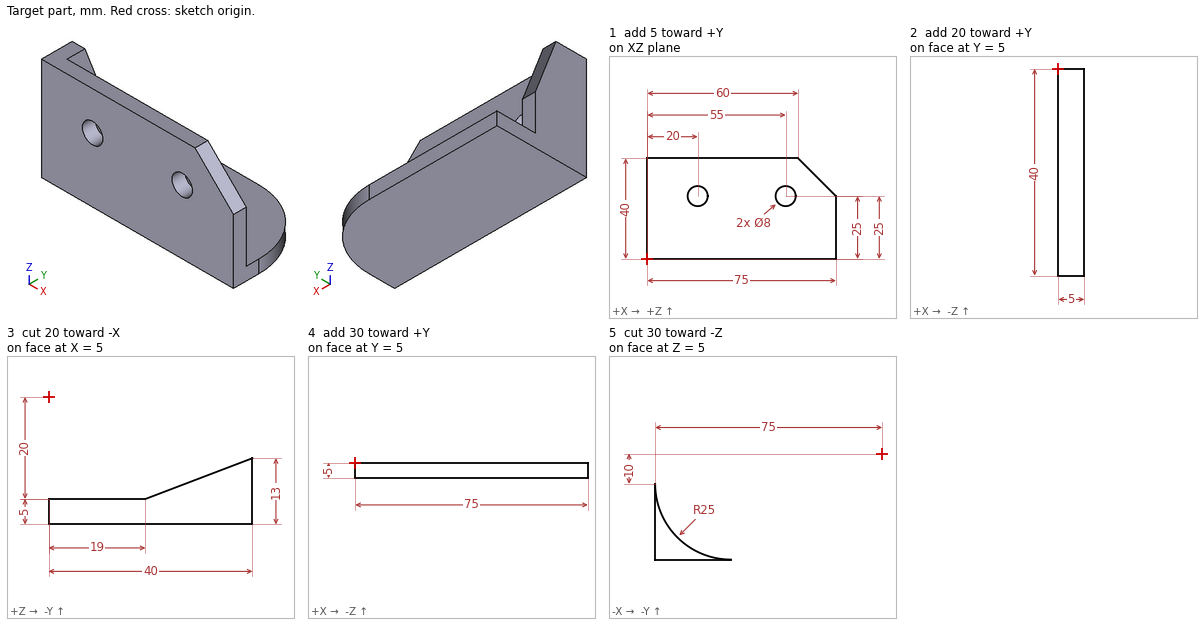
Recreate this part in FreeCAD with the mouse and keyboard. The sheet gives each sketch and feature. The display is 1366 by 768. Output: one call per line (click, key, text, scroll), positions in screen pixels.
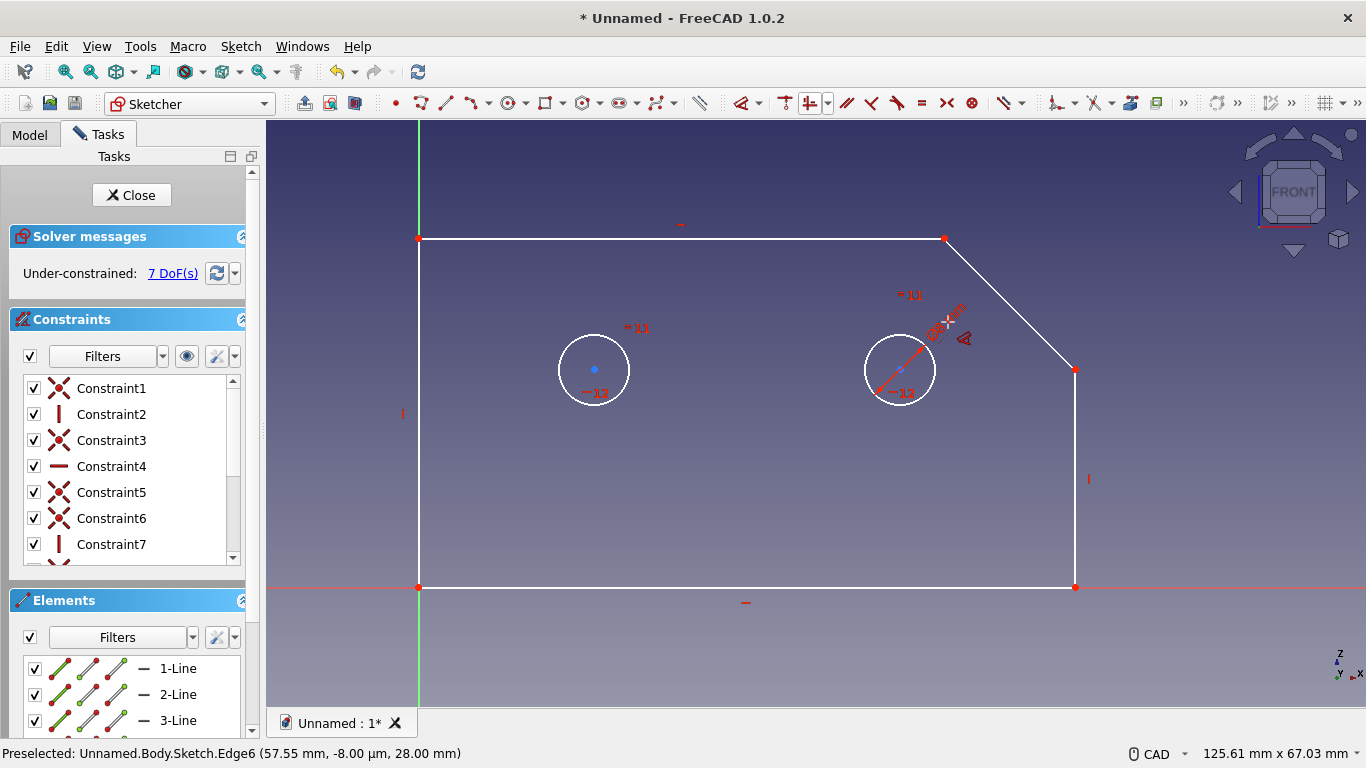
click(419, 483)
click(385, 413)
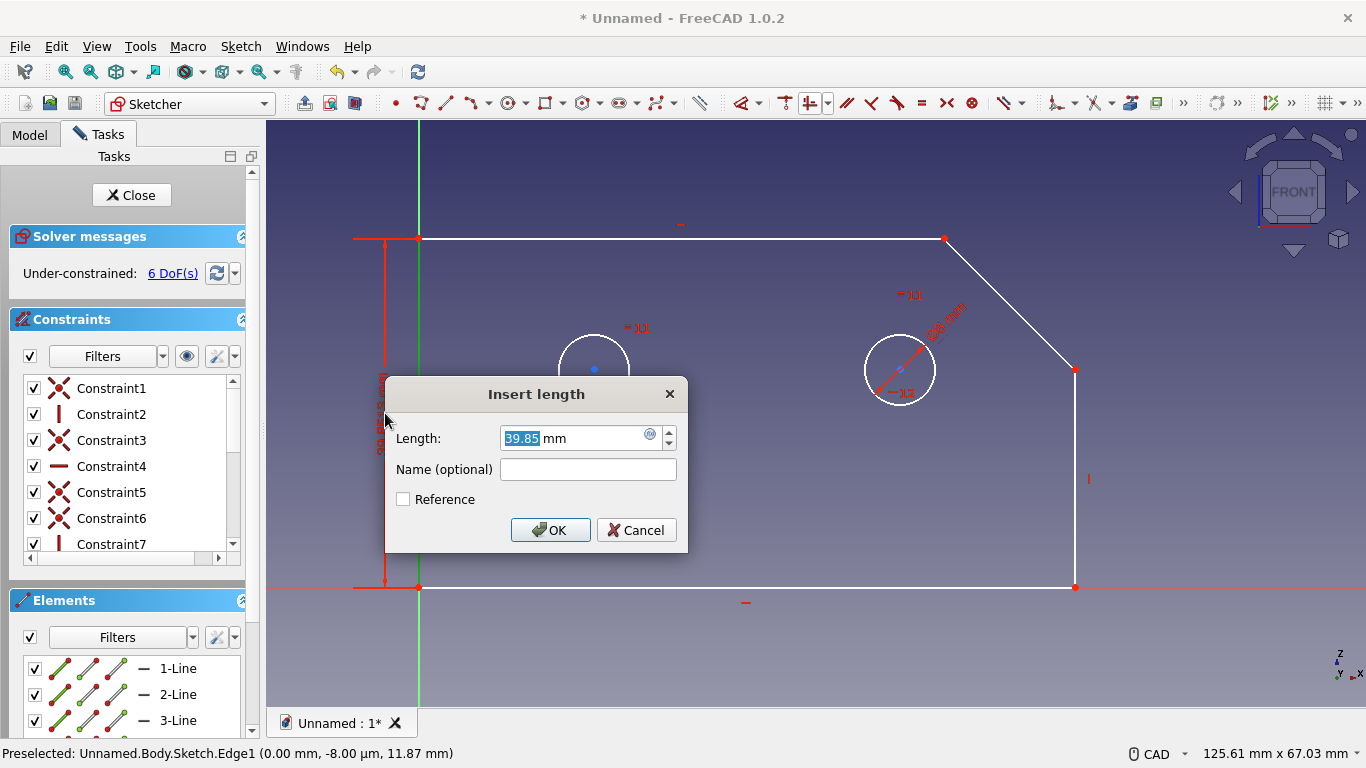
text(40)
key(Return)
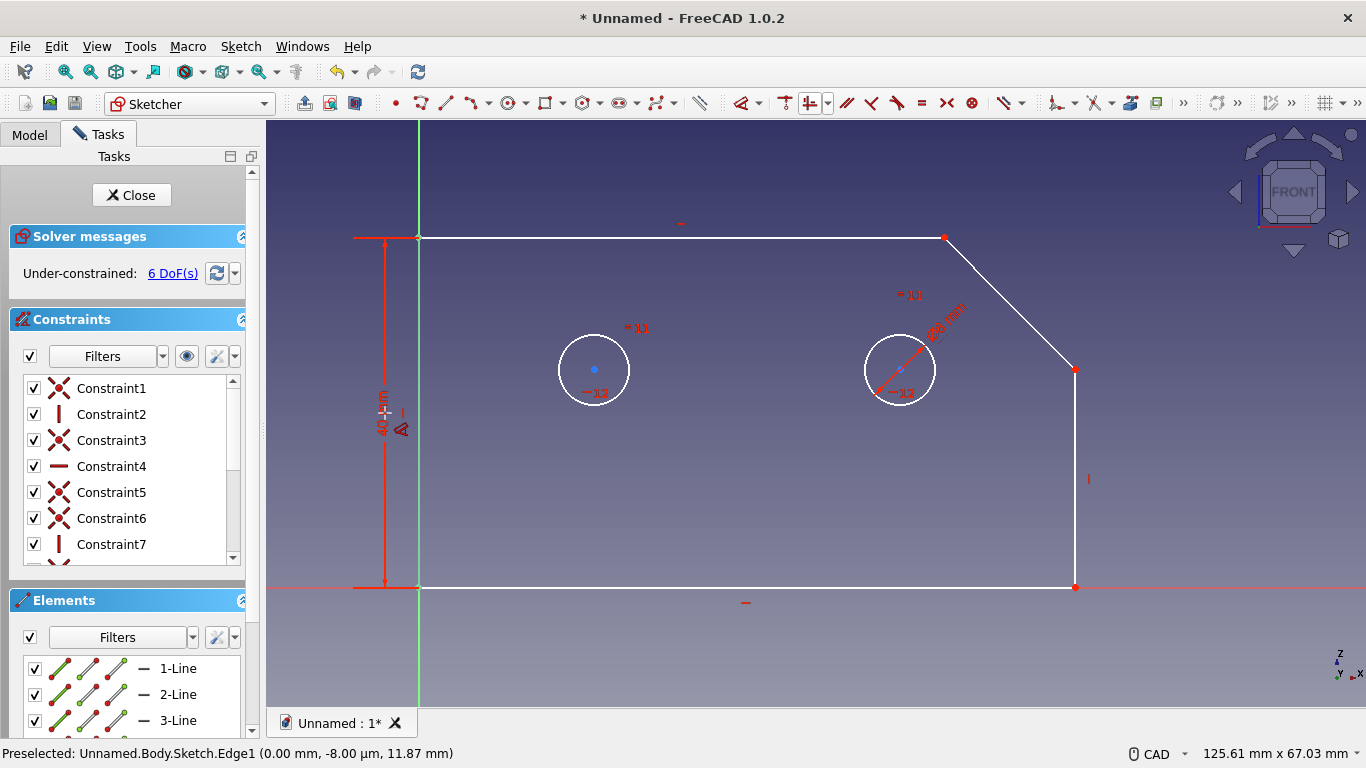
click(576, 238)
click(681, 204)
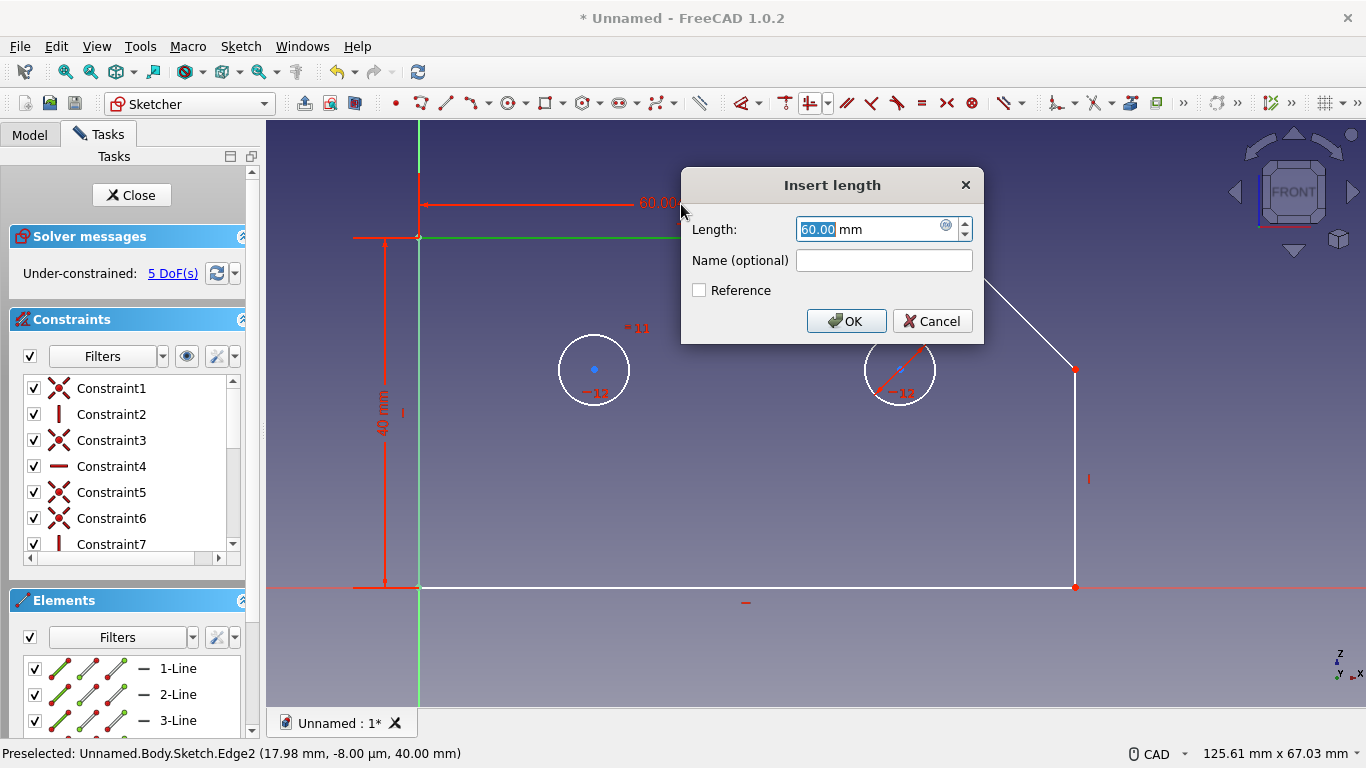
text(60)
key(Return)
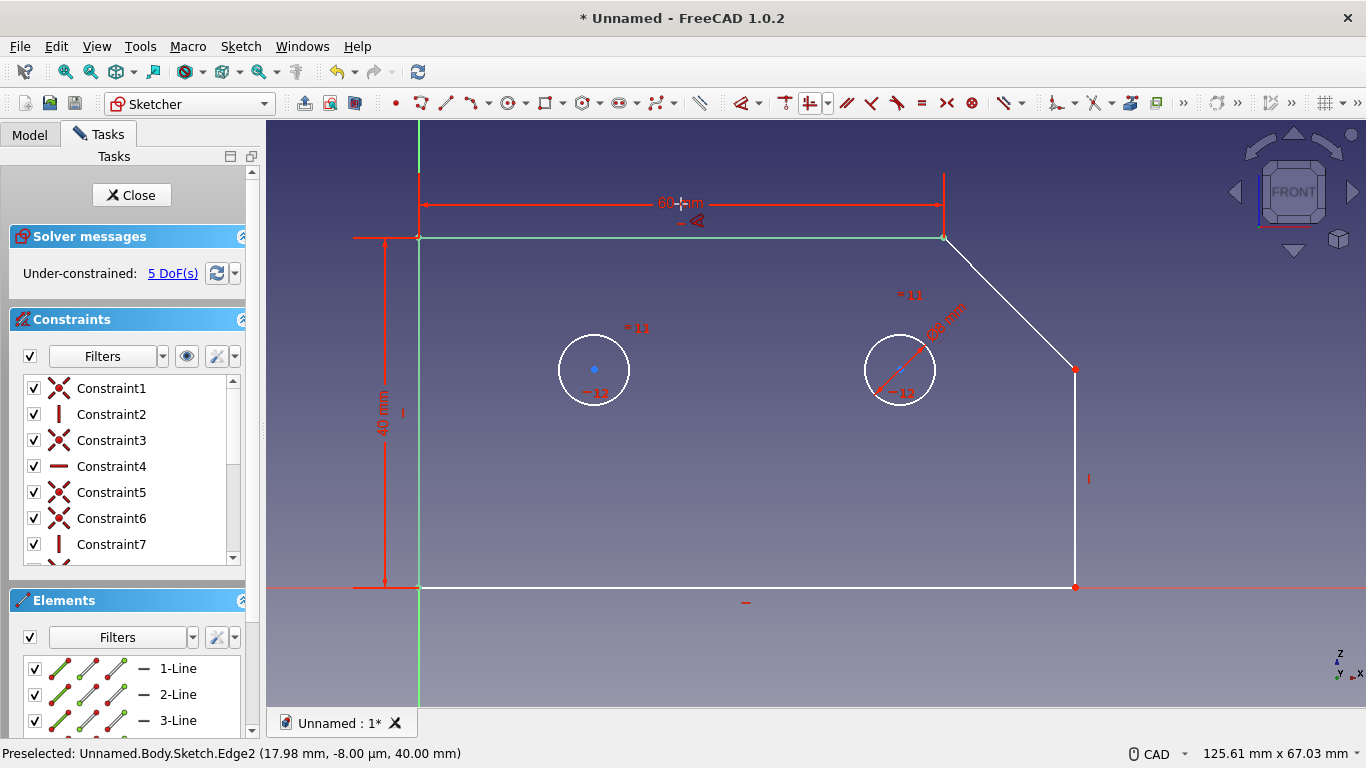
click(1075, 435)
click(1109, 479)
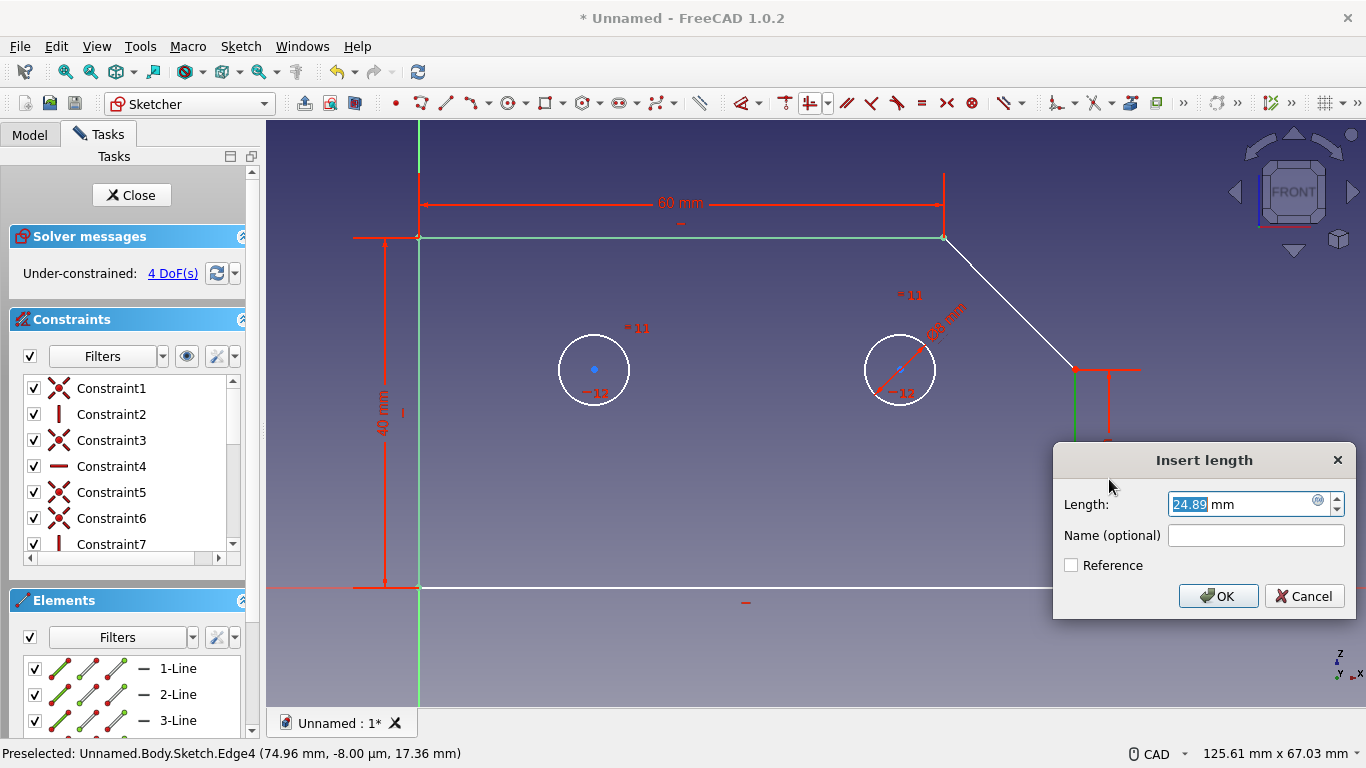
text(25)
key(Return)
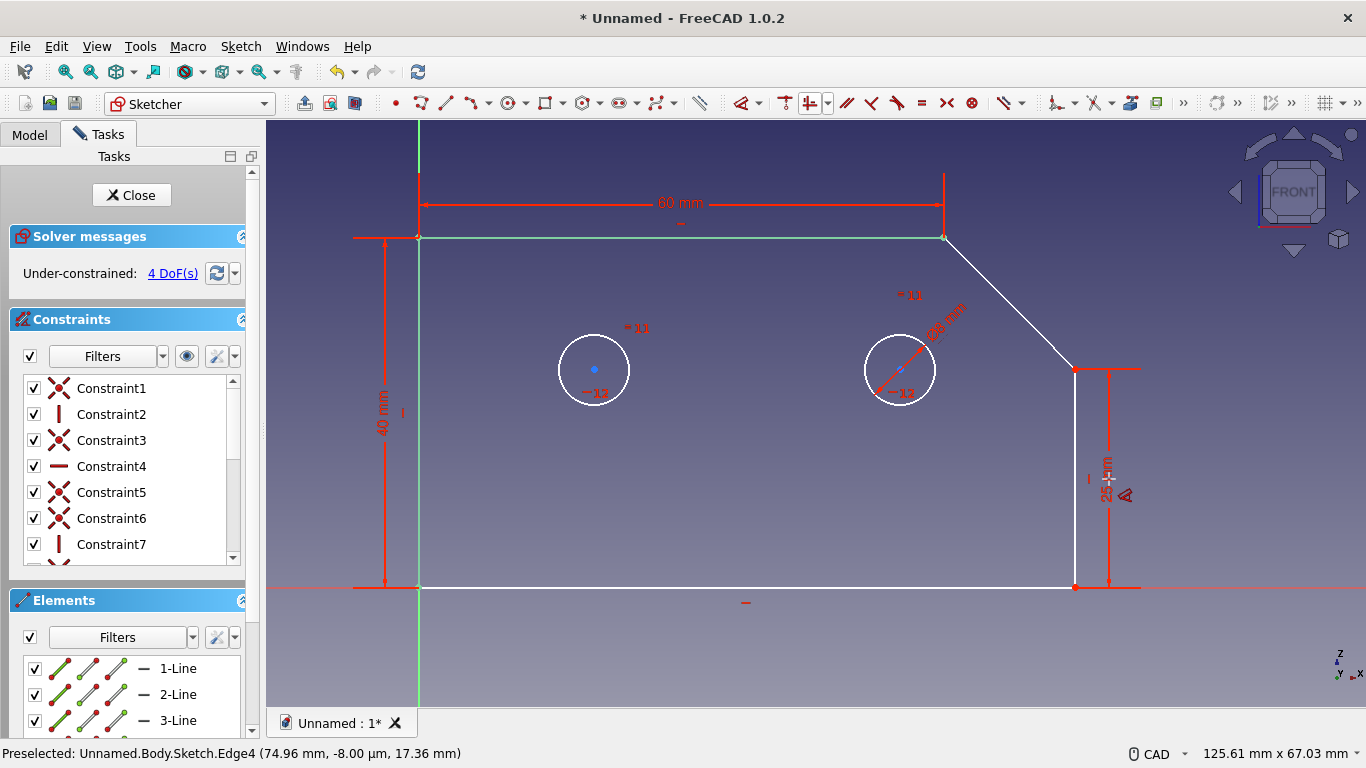
click(878, 588)
click(747, 622)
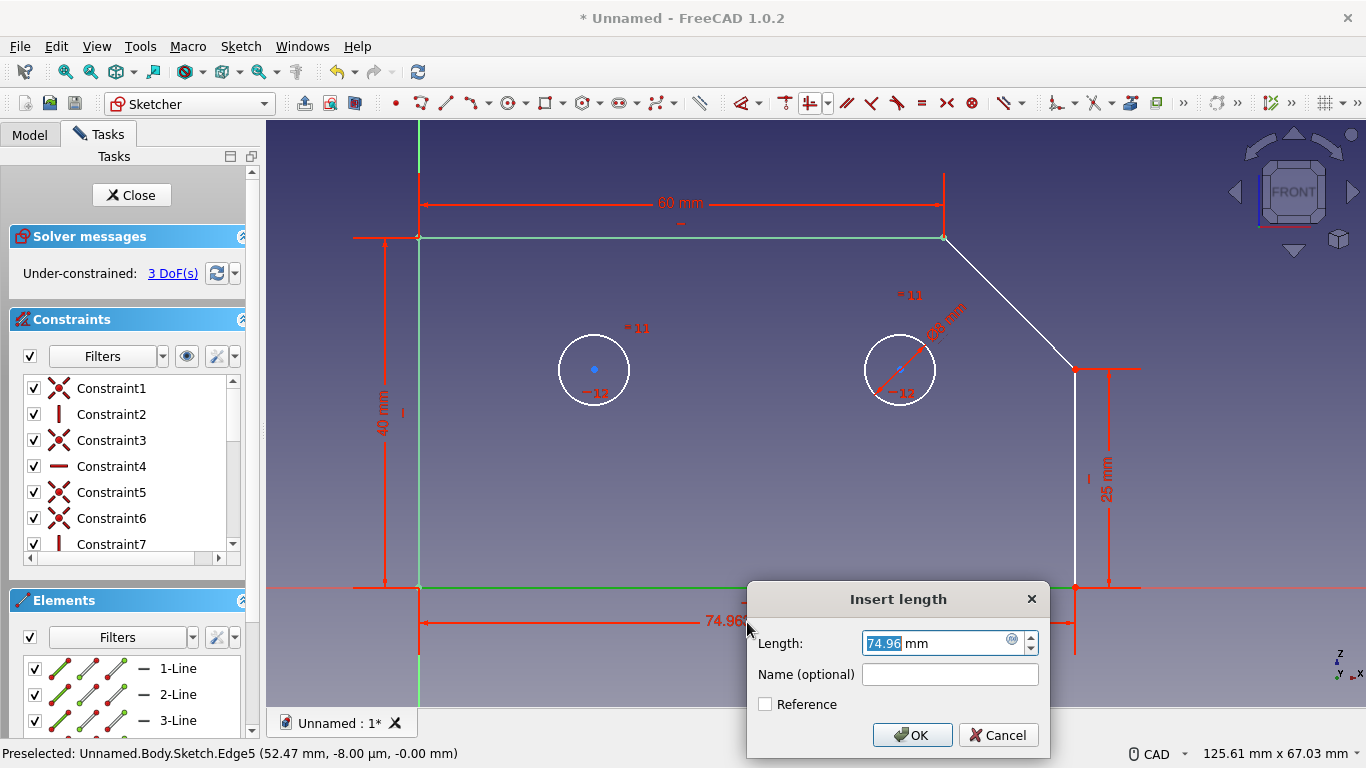
text(75)
key(Return)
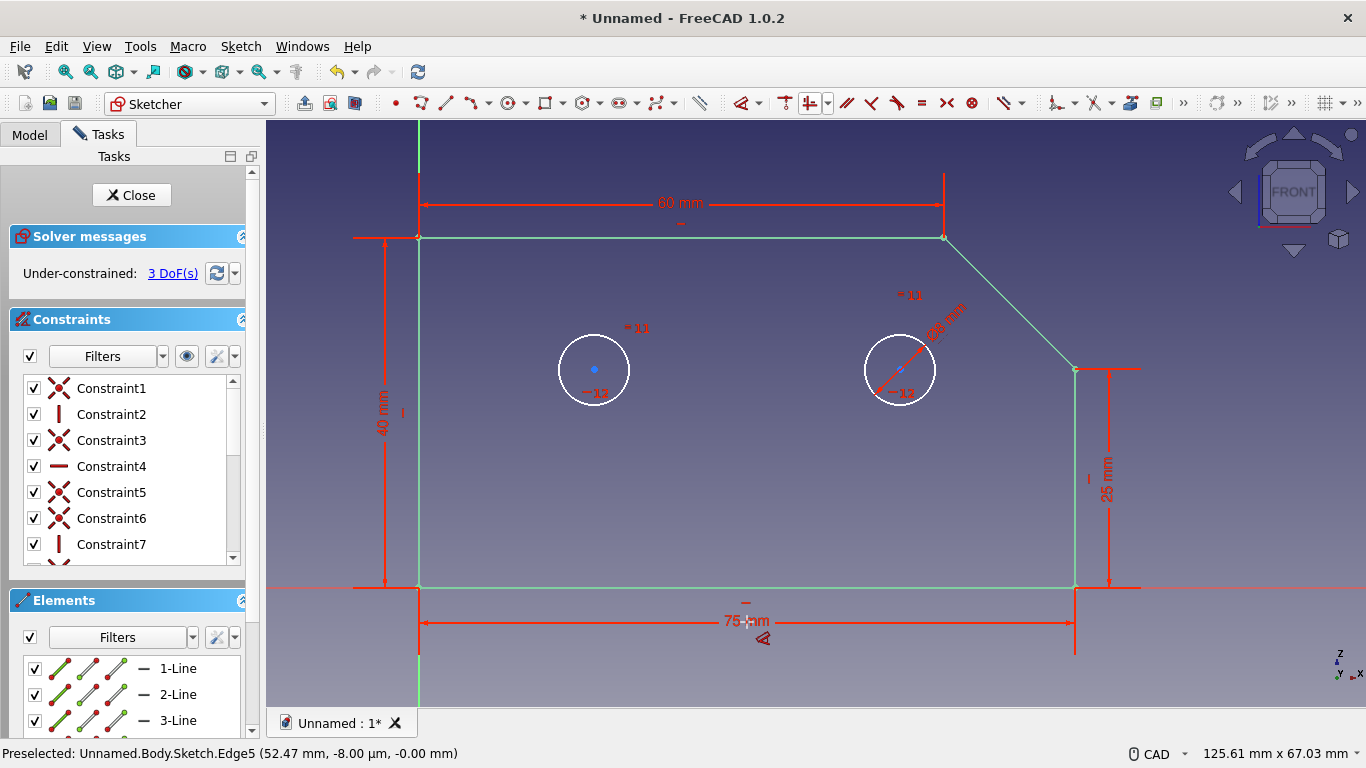
click(900, 370)
click(659, 622)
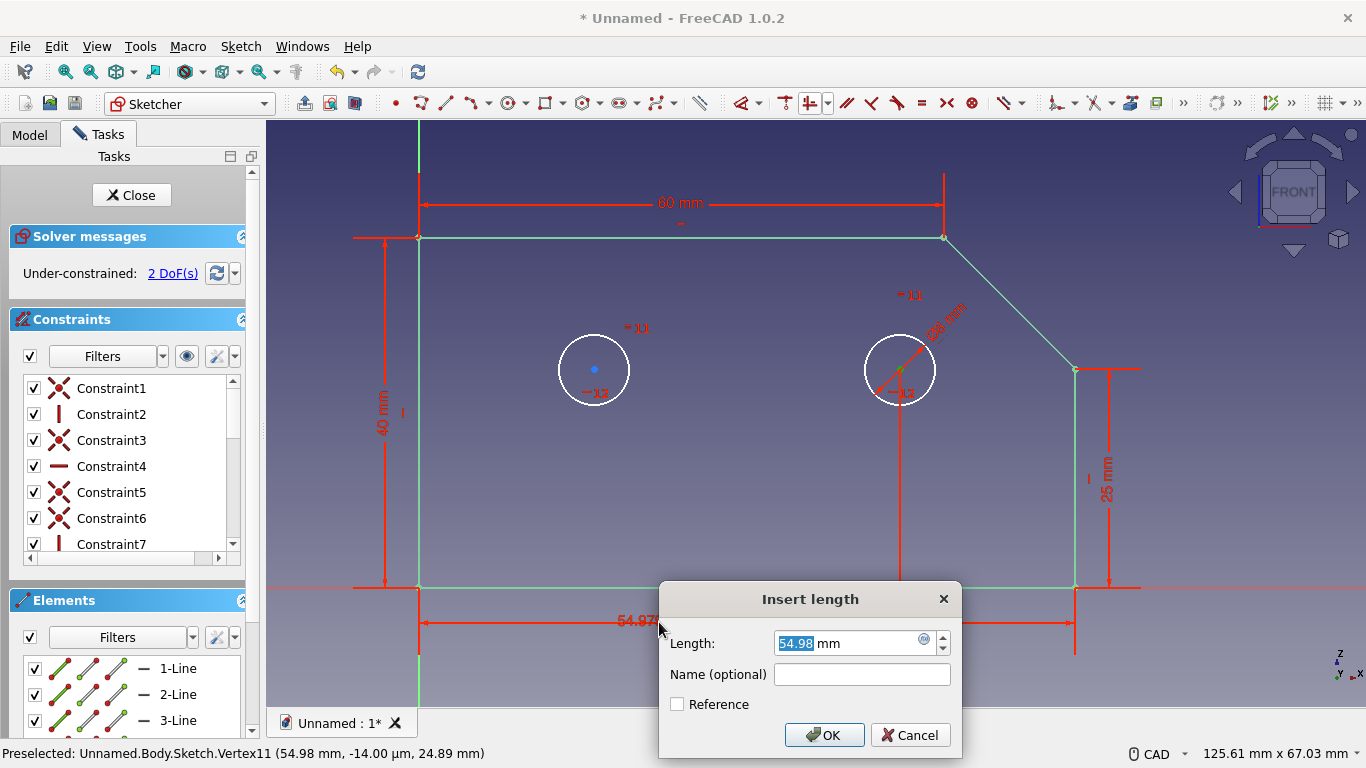
text(55)
key(Return)